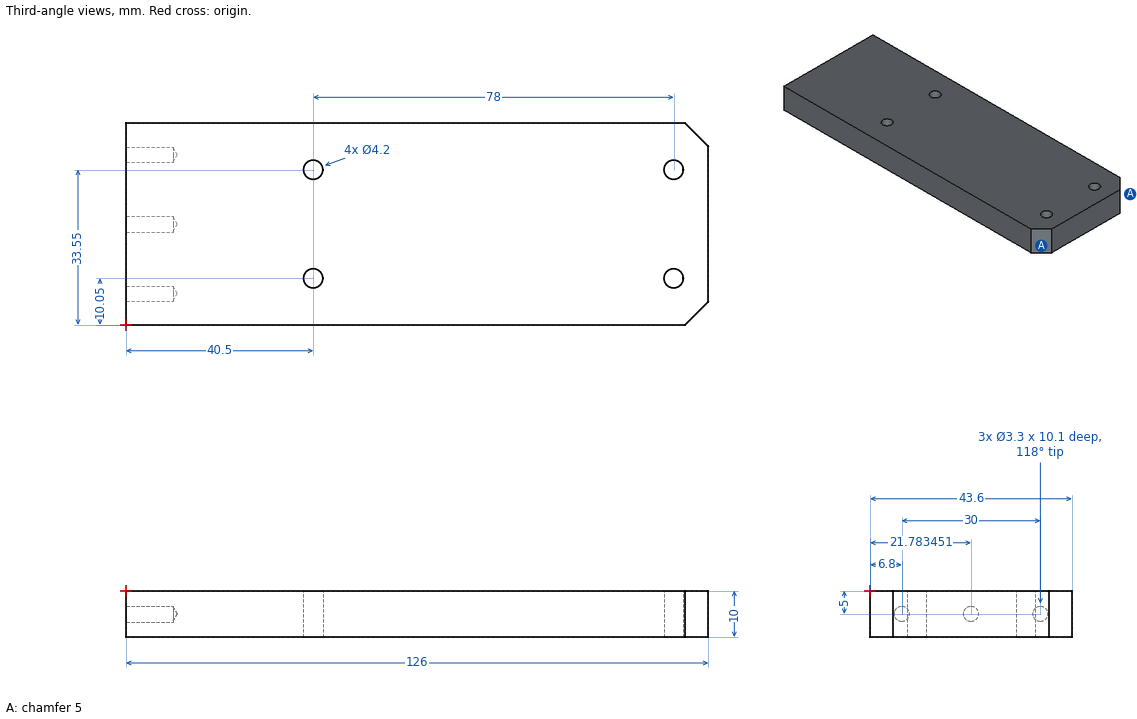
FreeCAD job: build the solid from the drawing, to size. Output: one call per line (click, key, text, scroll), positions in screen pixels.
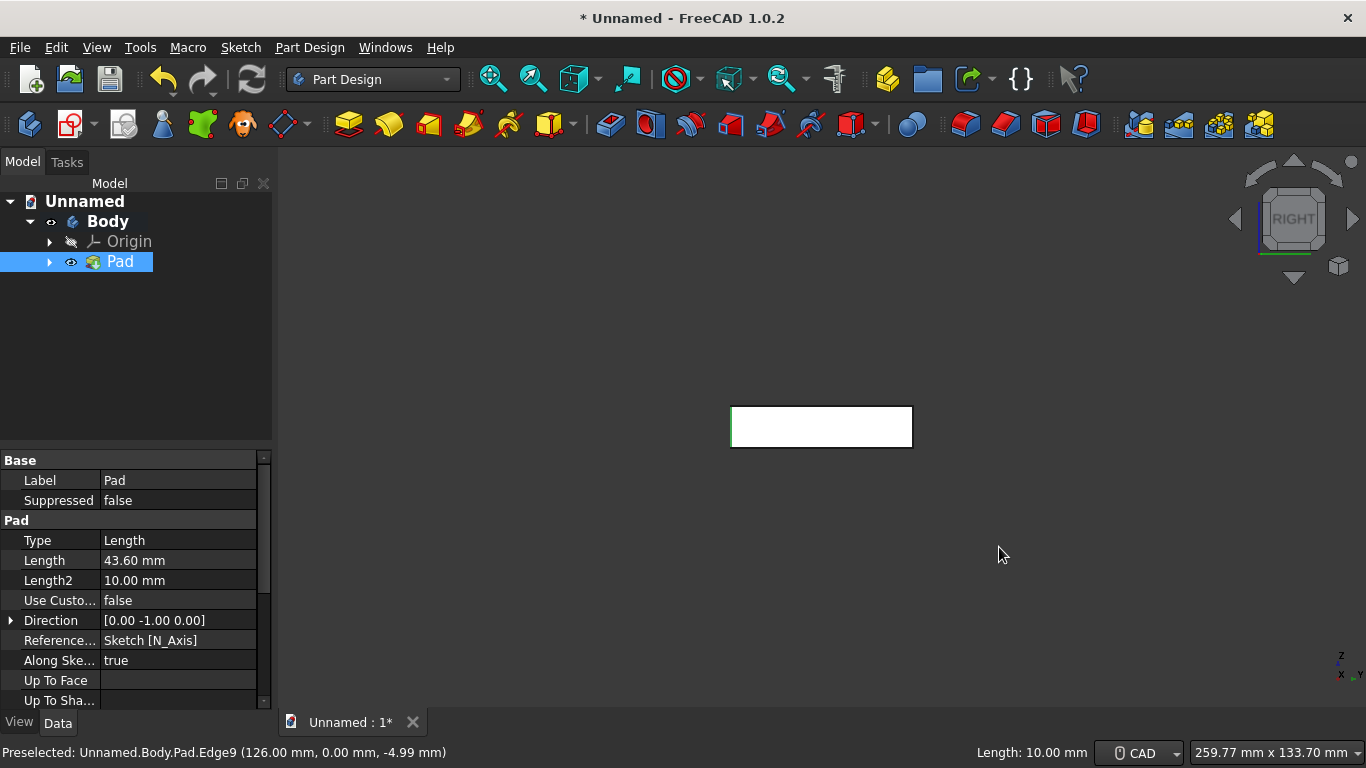
click(494, 80)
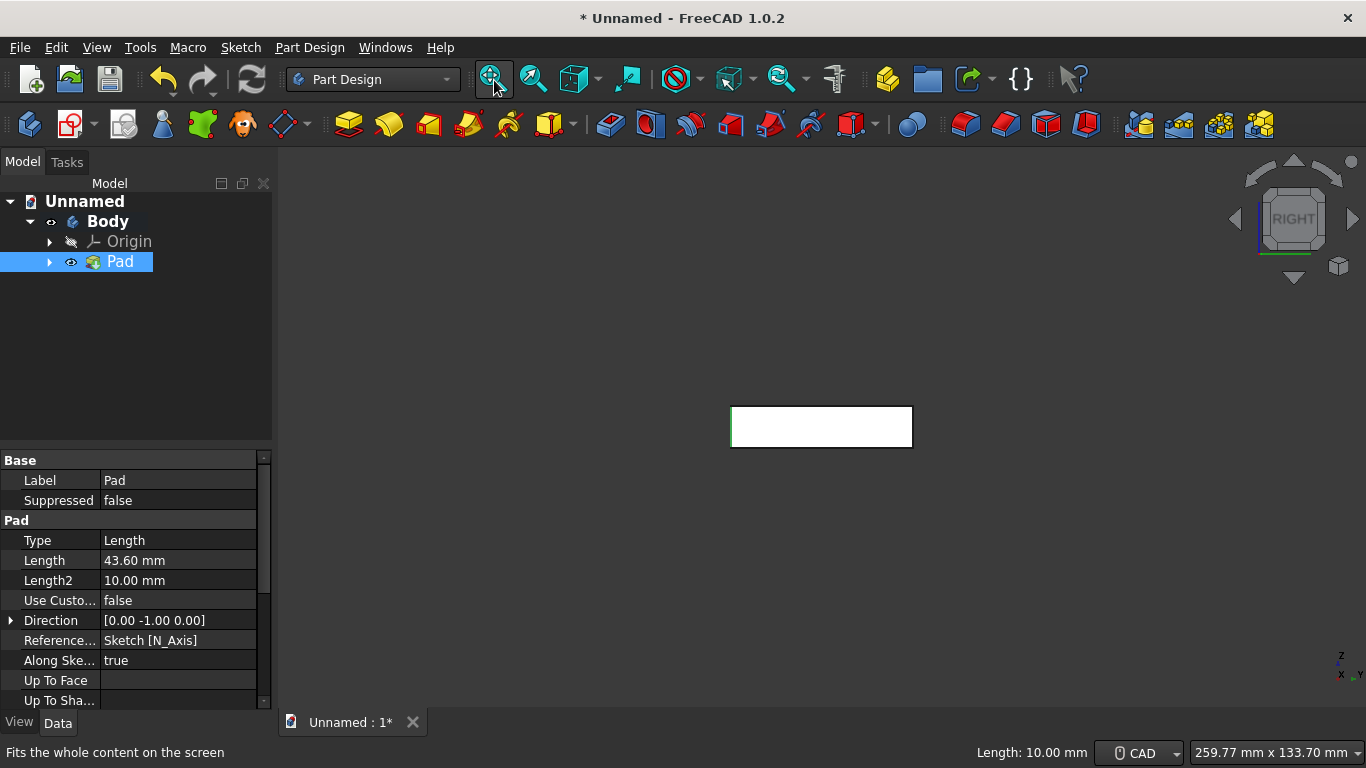
click(913, 426, ctrl)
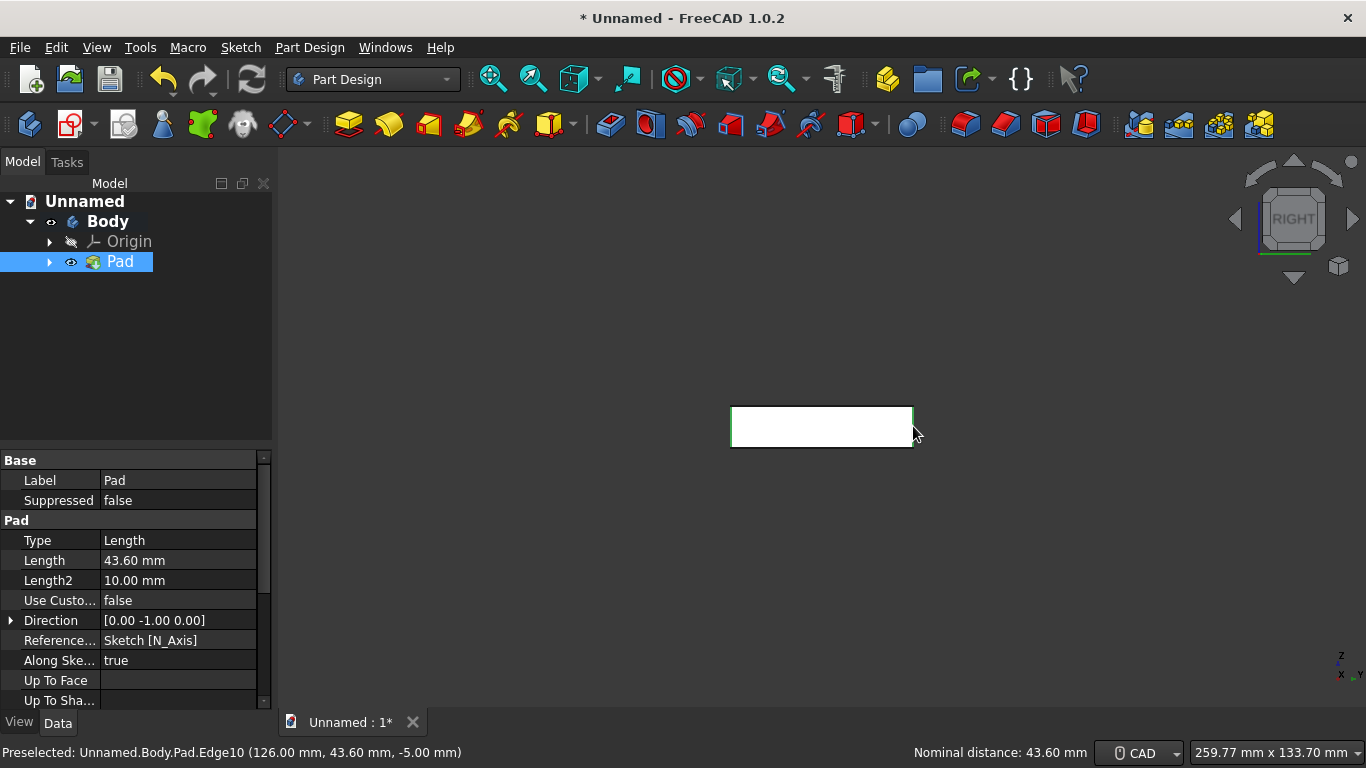
click(1006, 124)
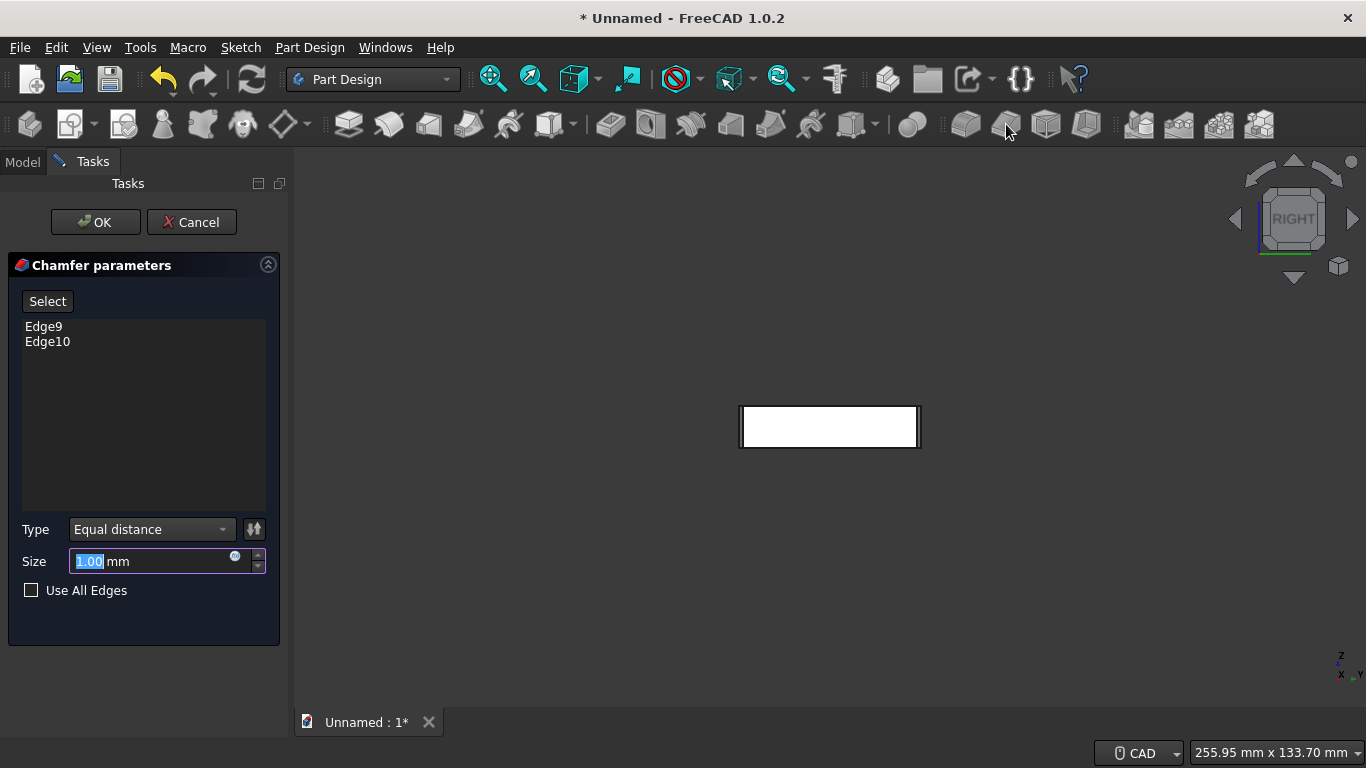
text(5)
key(Tab)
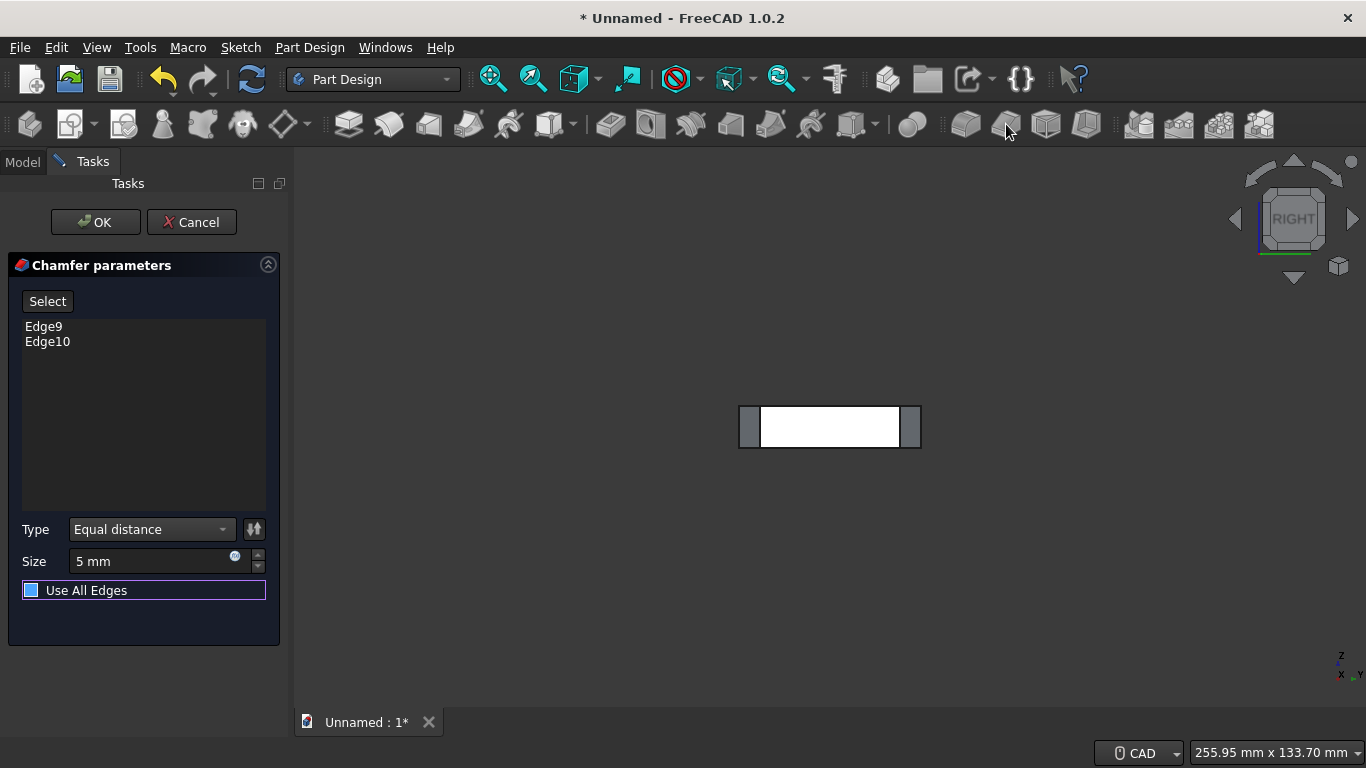
click(96, 222)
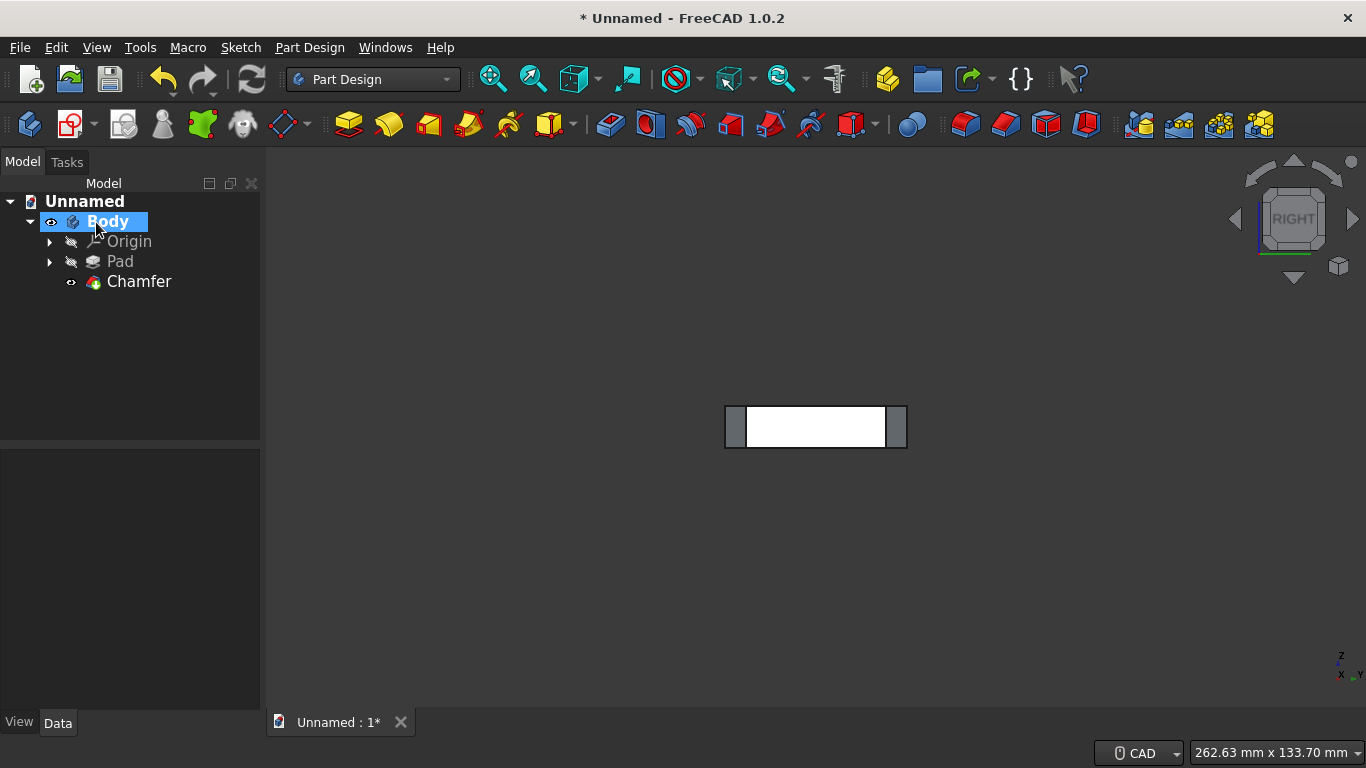
click(494, 80)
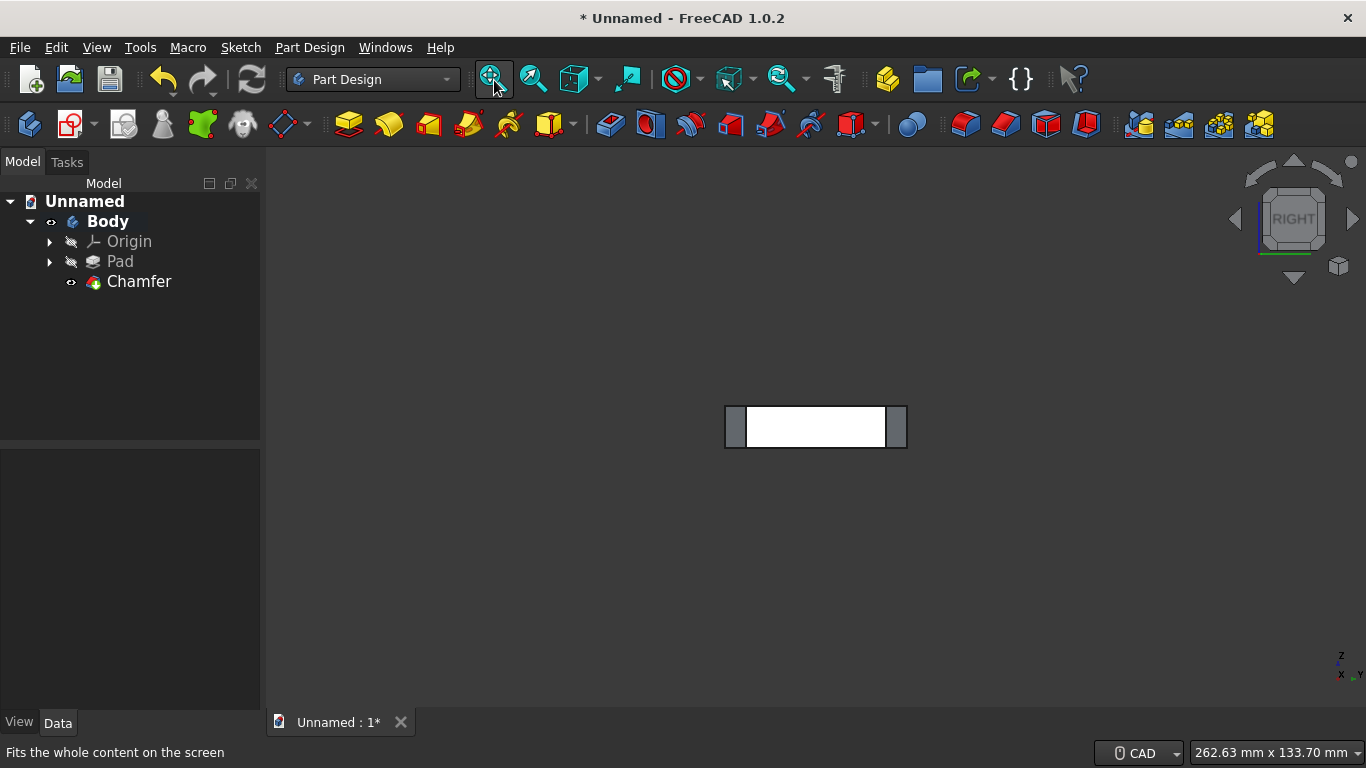
click(70, 124)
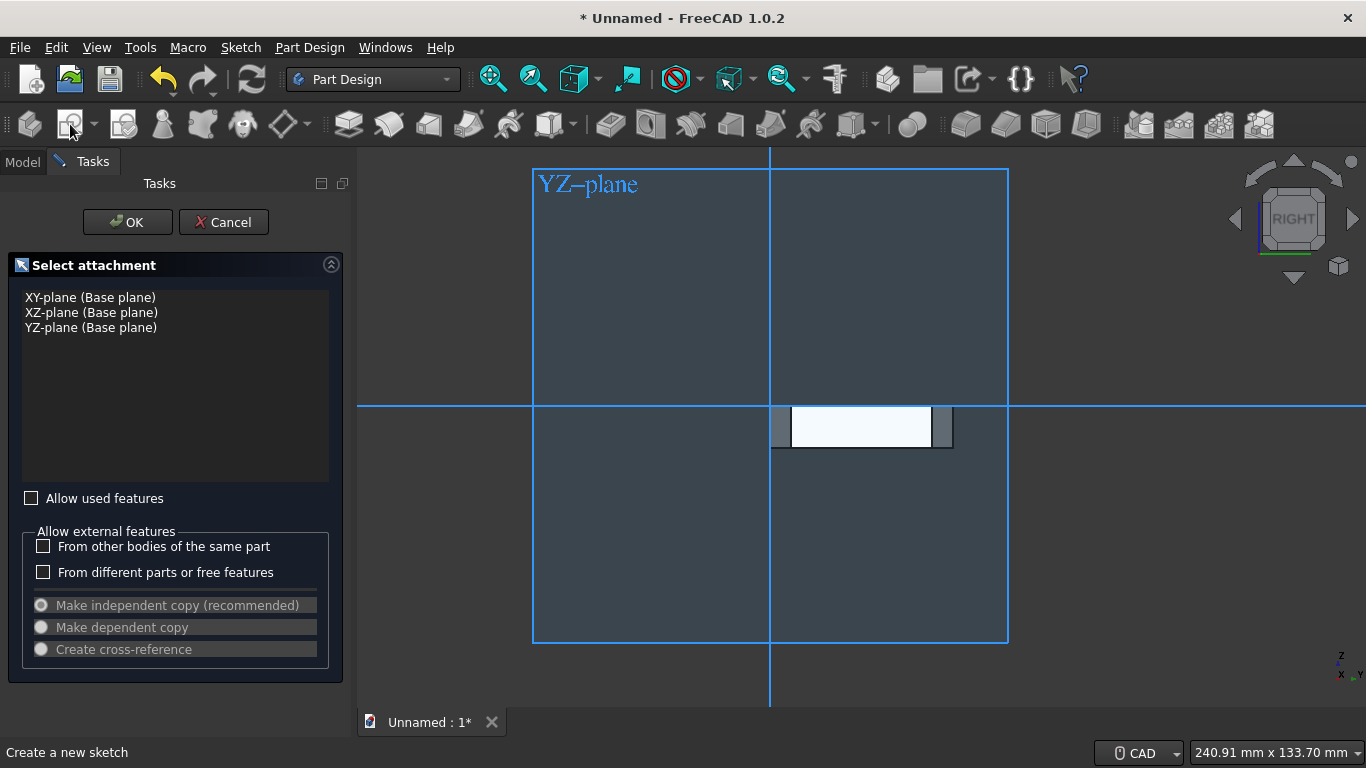
click(82, 328)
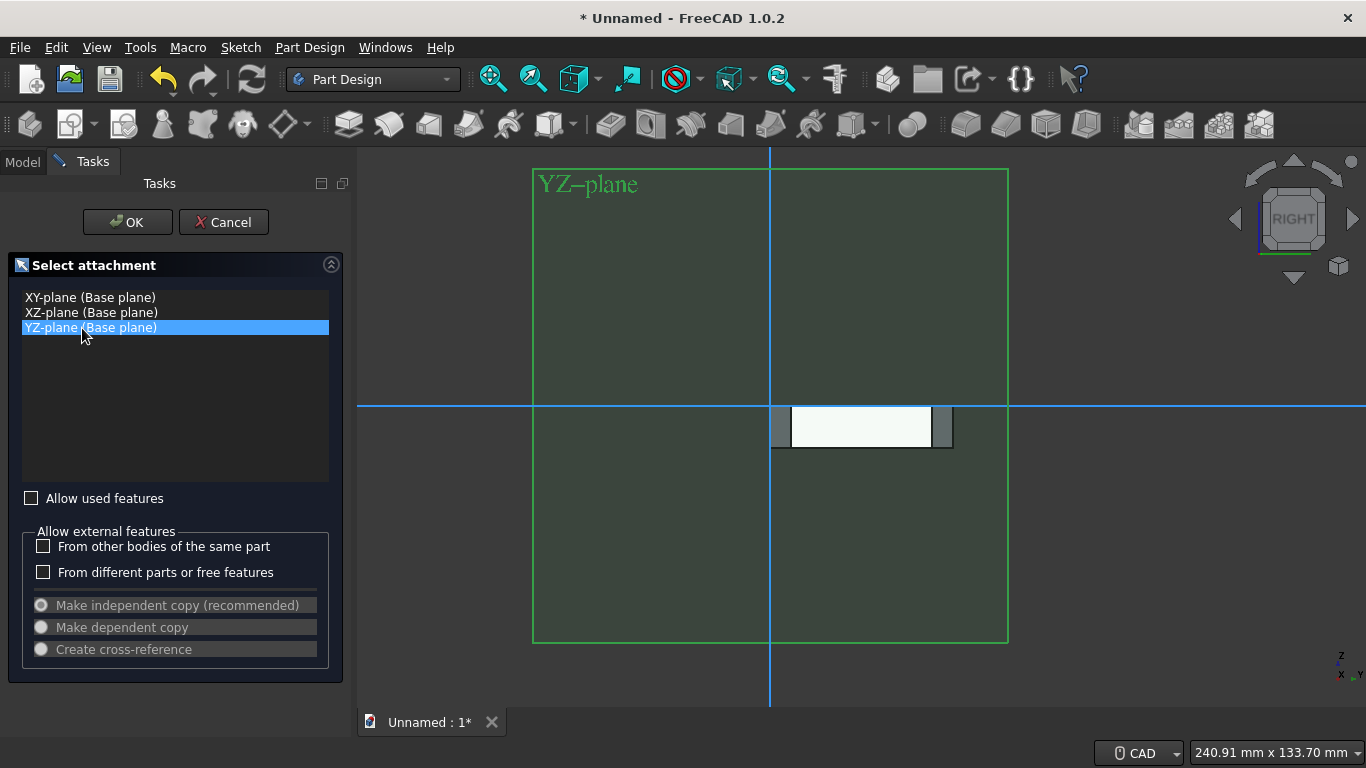
click(128, 222)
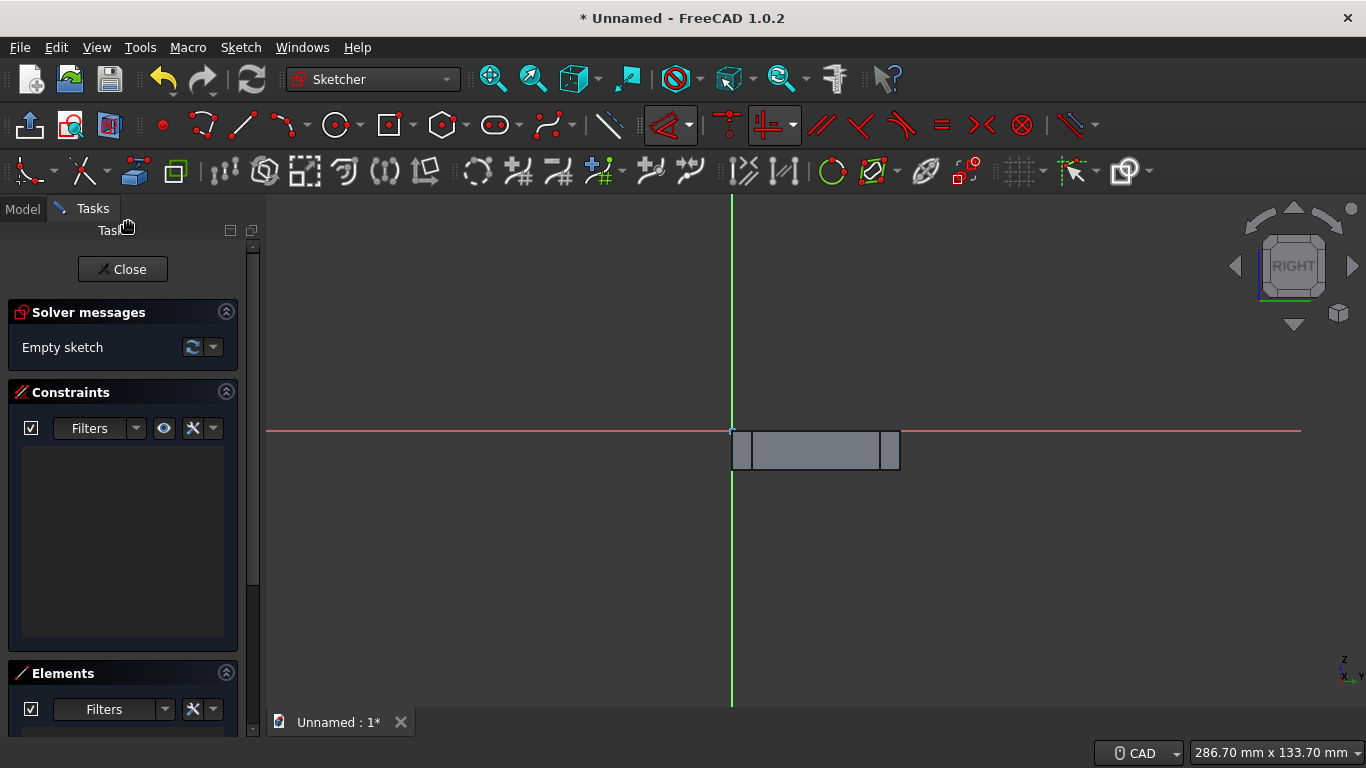
click(110, 126)